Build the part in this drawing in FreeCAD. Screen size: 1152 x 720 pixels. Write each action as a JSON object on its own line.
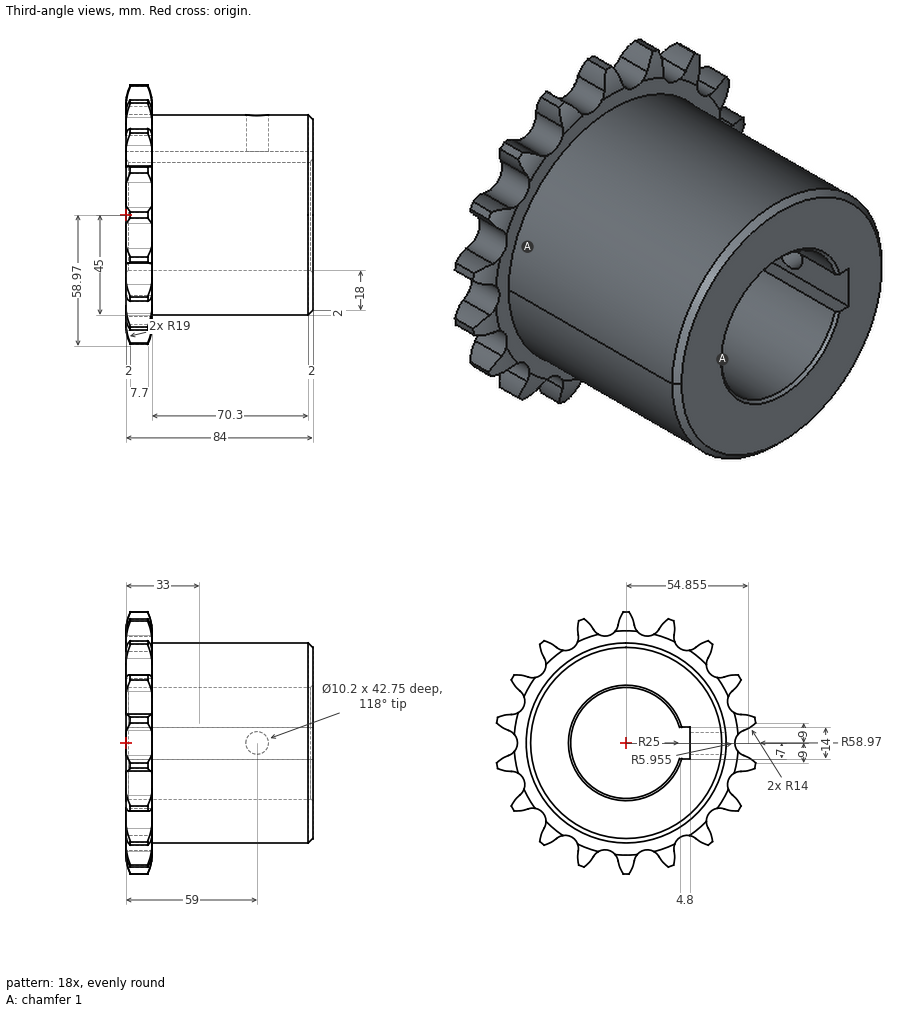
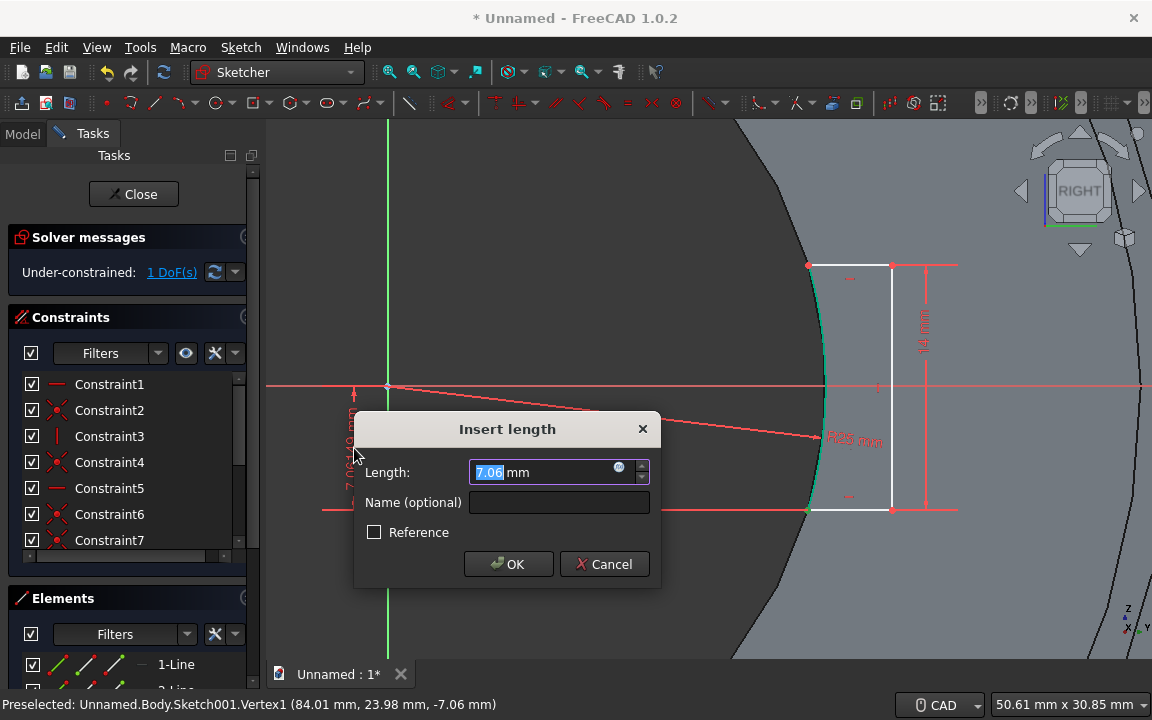
{"action": "type", "text": "7"}
{"action": "key", "text": "Return"}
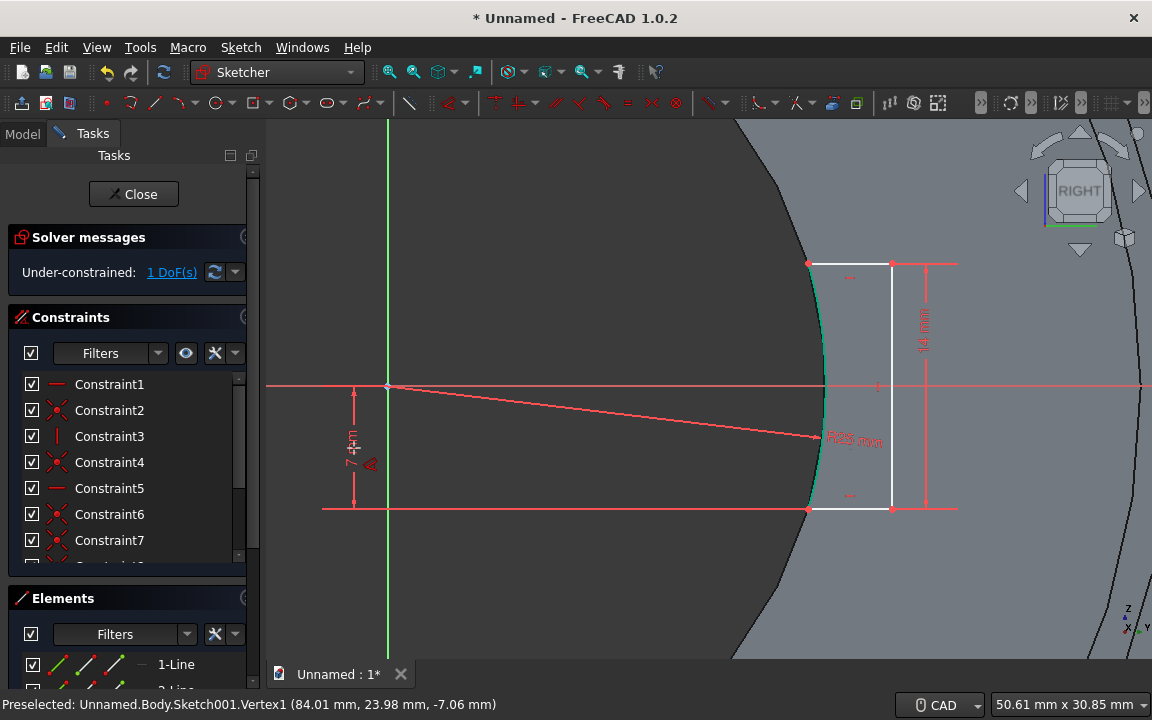
{"action": "left_click", "coordinate": [833, 509]}
{"action": "left_click", "coordinate": [850, 543]}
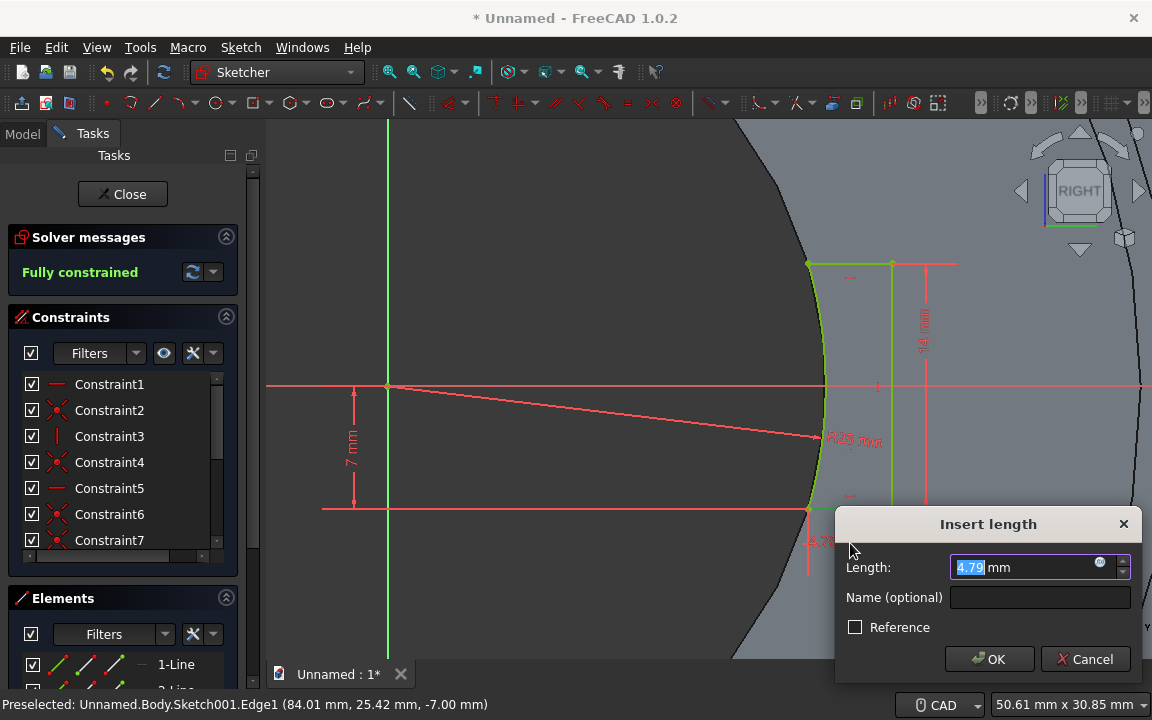
{"action": "type", "text": "4.8"}
{"action": "key", "text": "Return"}
{"action": "key", "text": "Escape"}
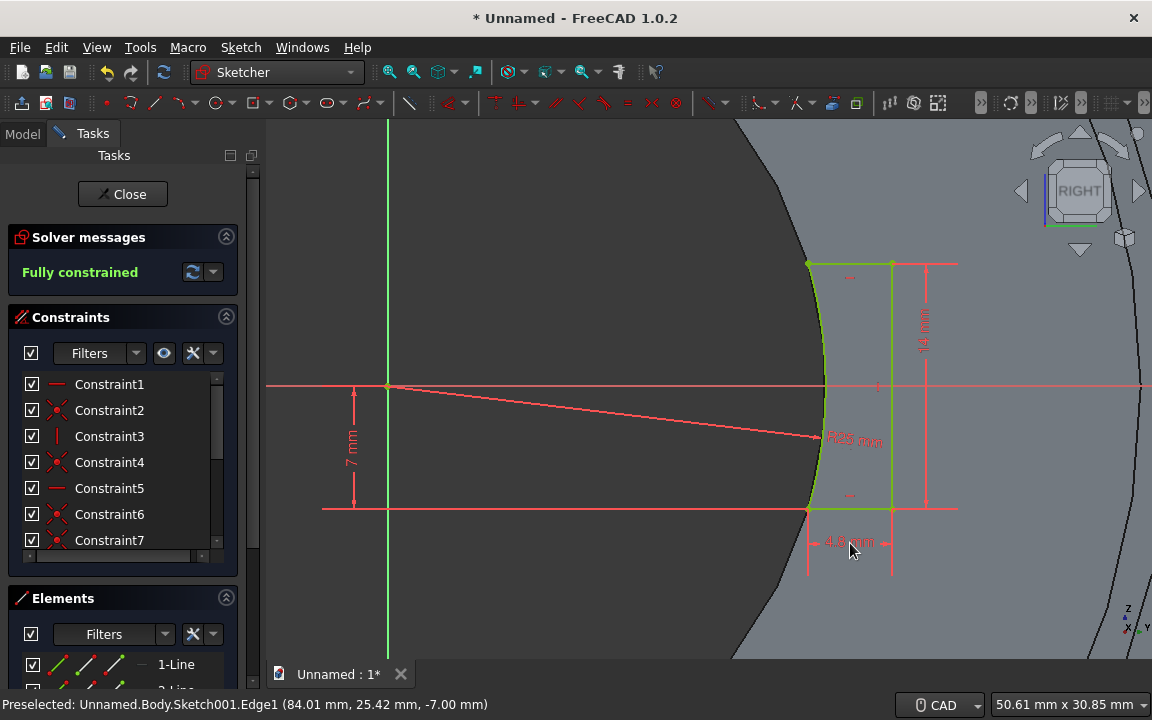
{"action": "left_click", "coordinate": [123, 194]}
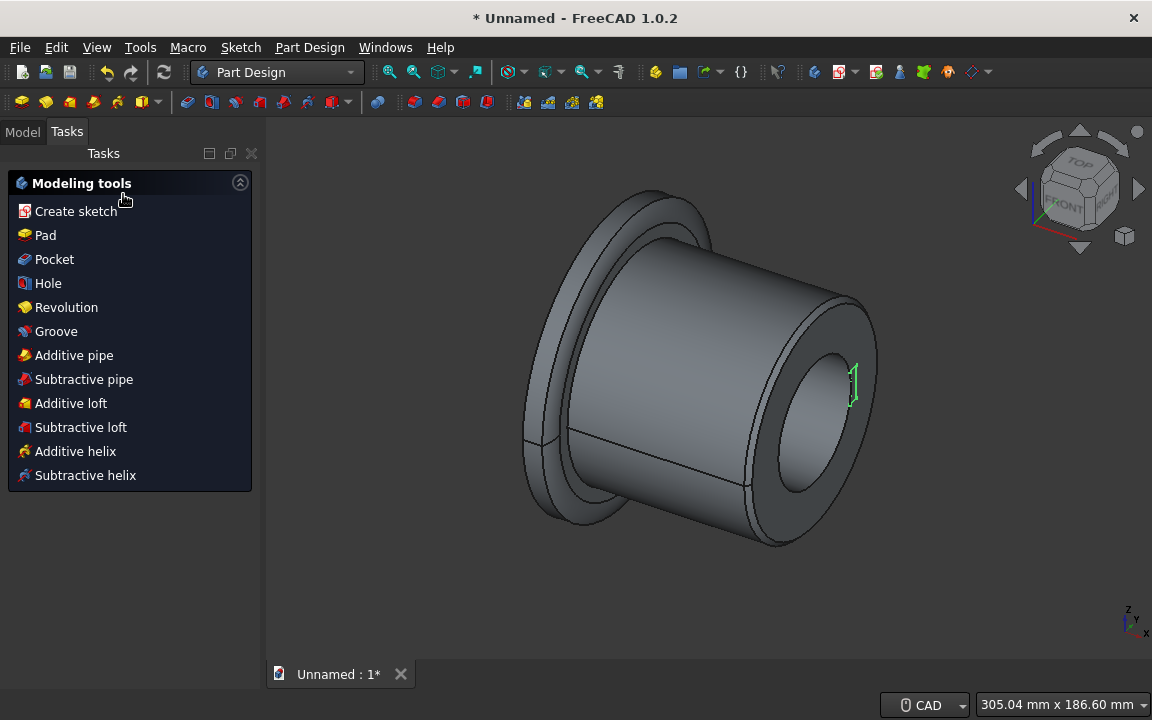
{"action": "left_click", "coordinate": [188, 102]}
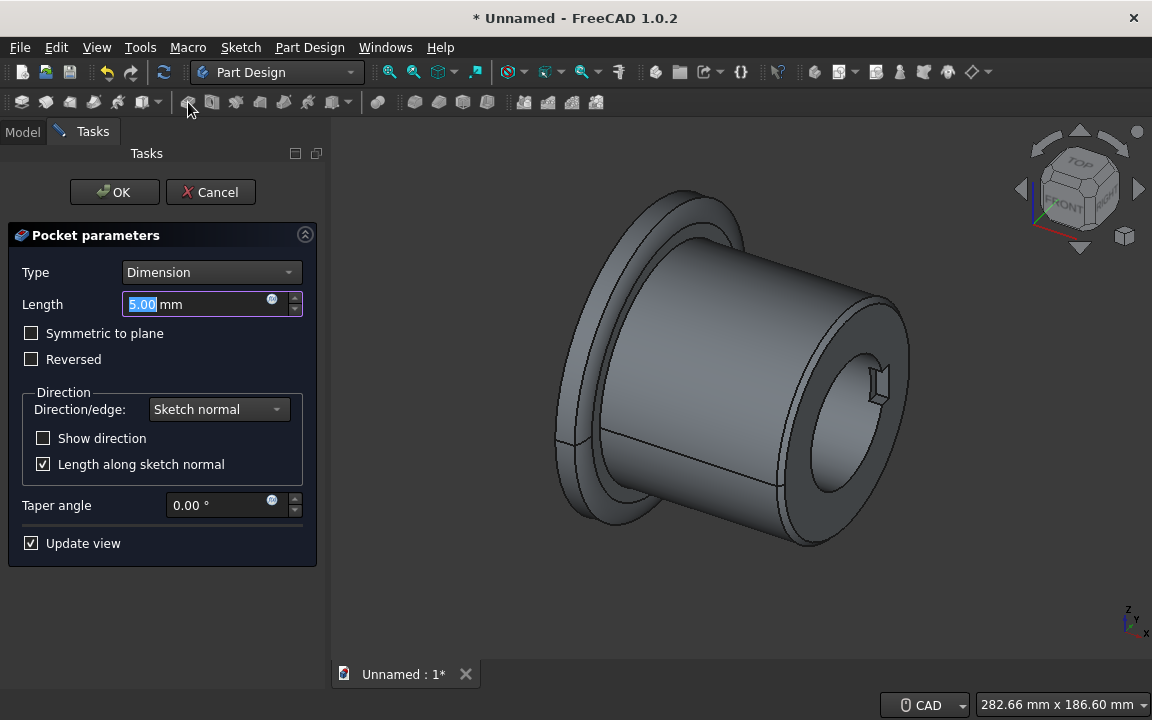
{"action": "left_click", "coordinate": [212, 272]}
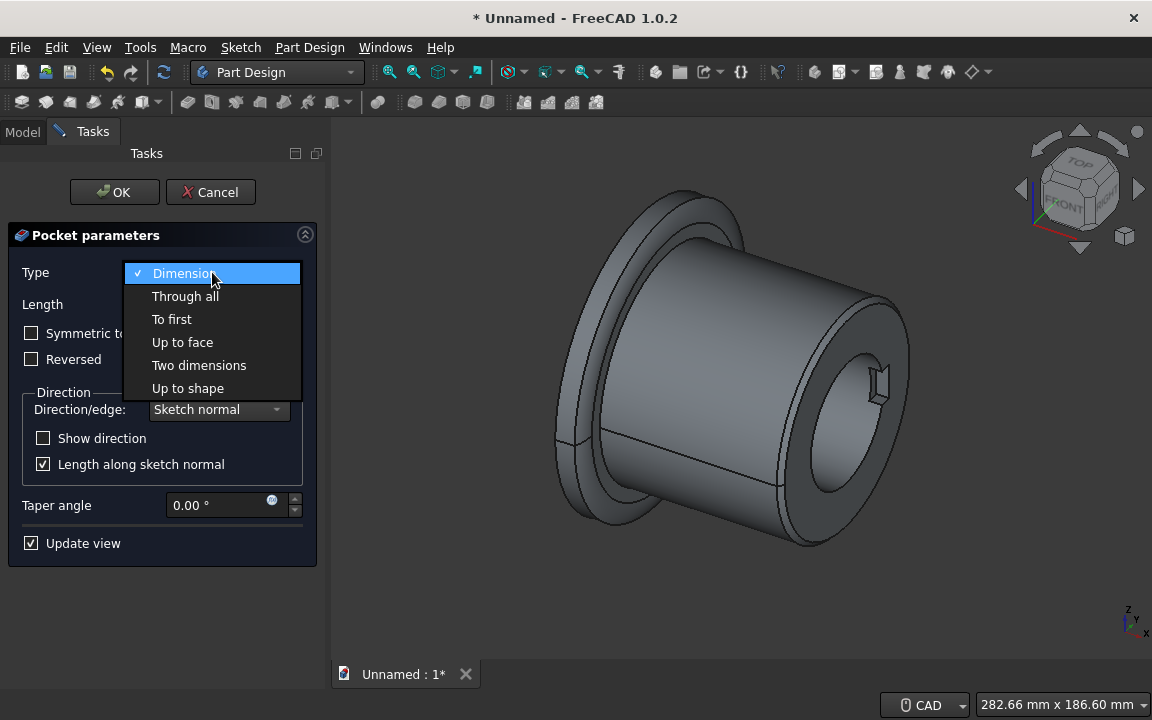
{"action": "left_click", "coordinate": [212, 296]}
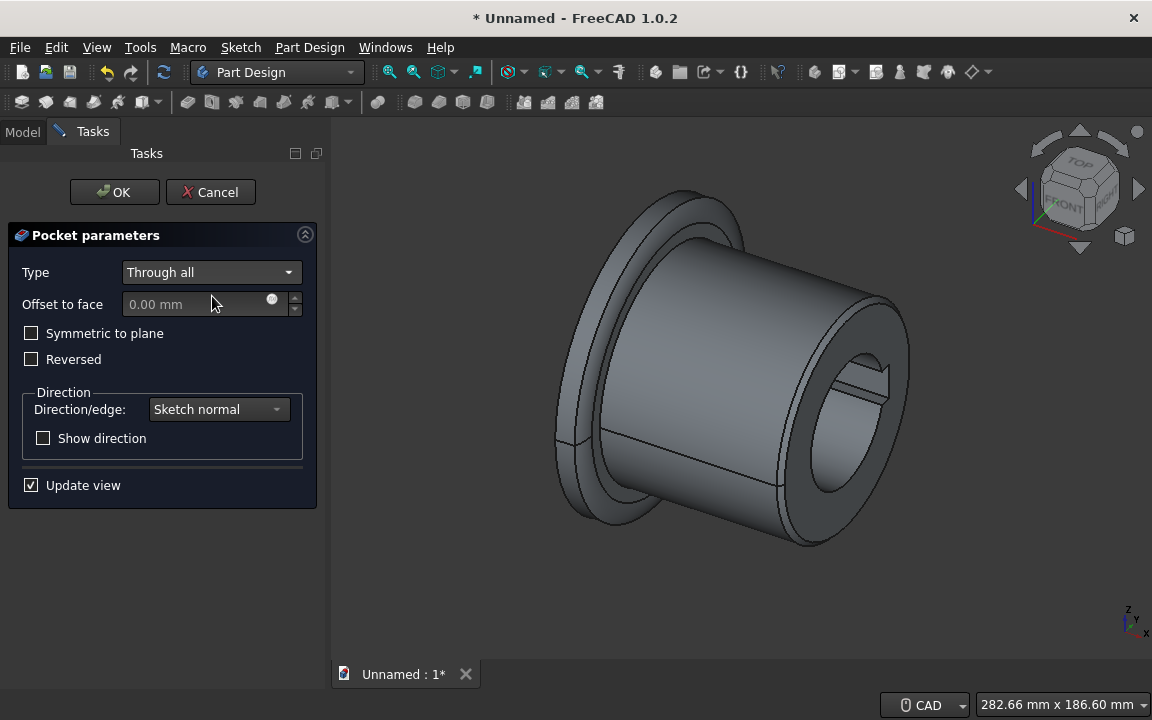
{"action": "left_click", "coordinate": [115, 192]}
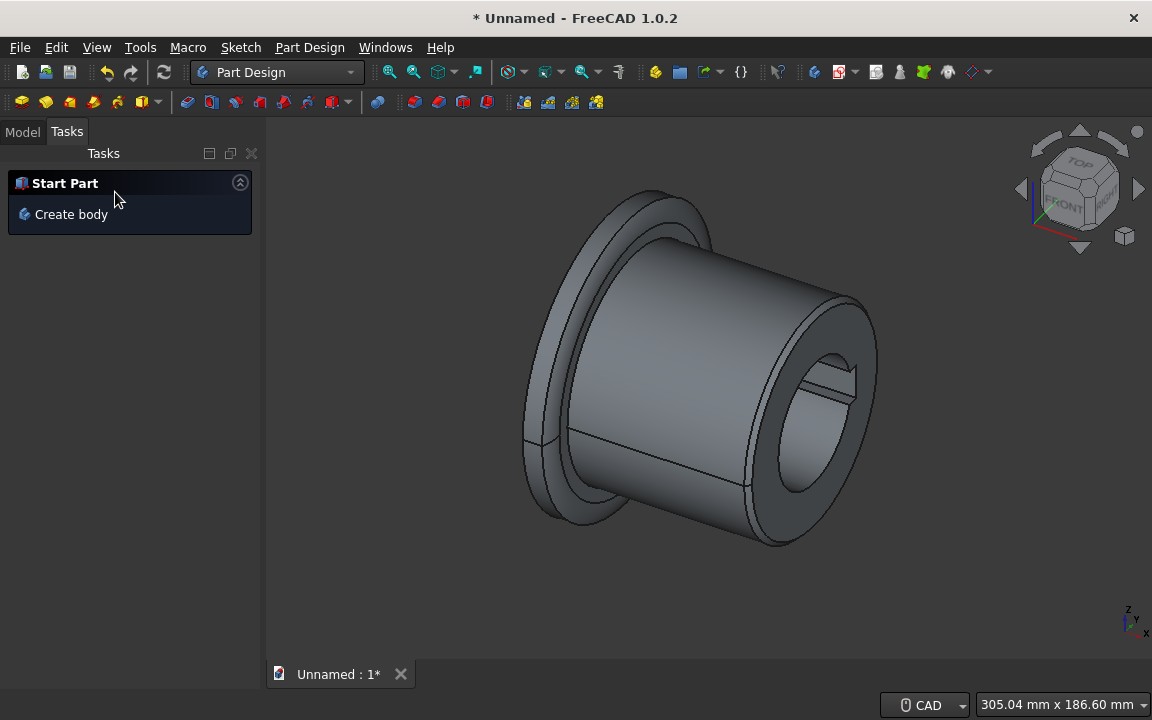
{"action": "left_click", "coordinate": [23, 131]}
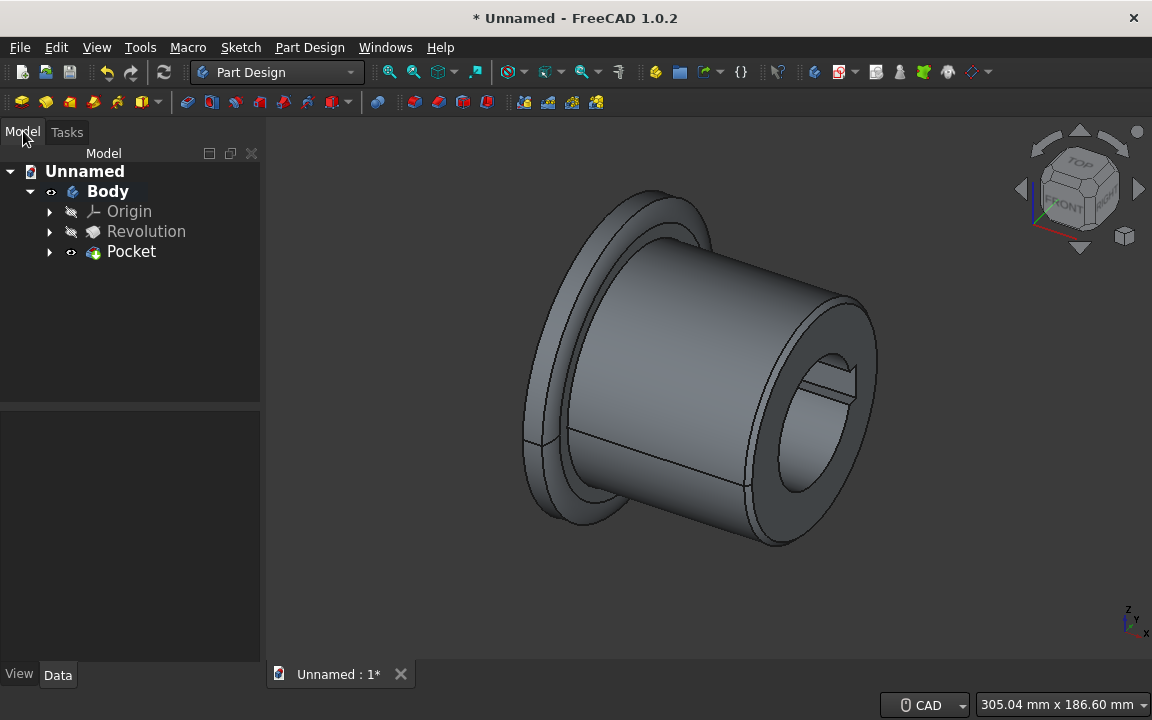
{"action": "left_click", "coordinate": [50, 212]}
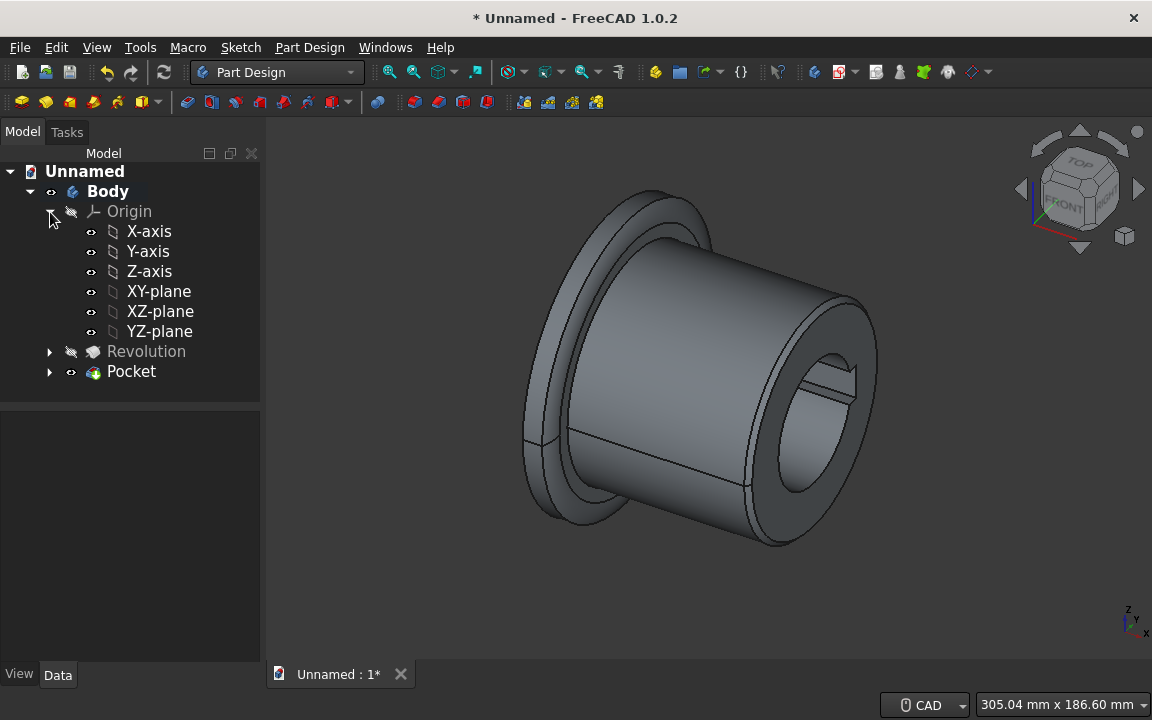
{"action": "left_click", "coordinate": [136, 312]}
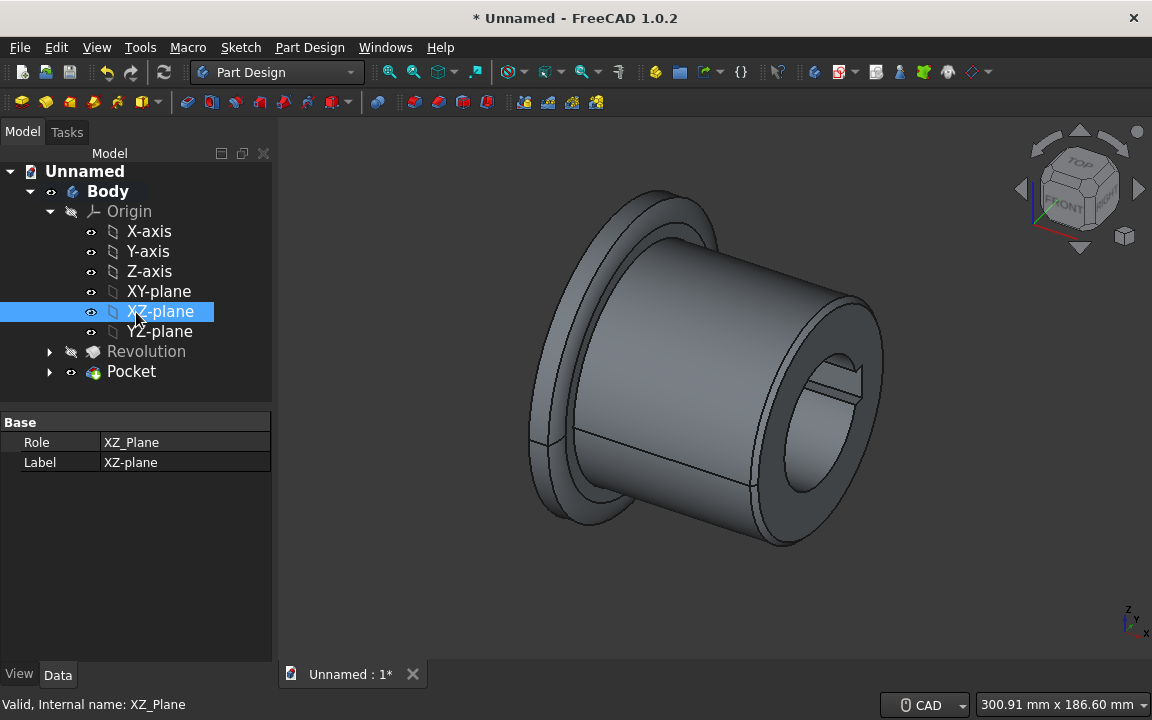
{"action": "left_click", "coordinate": [972, 72]}